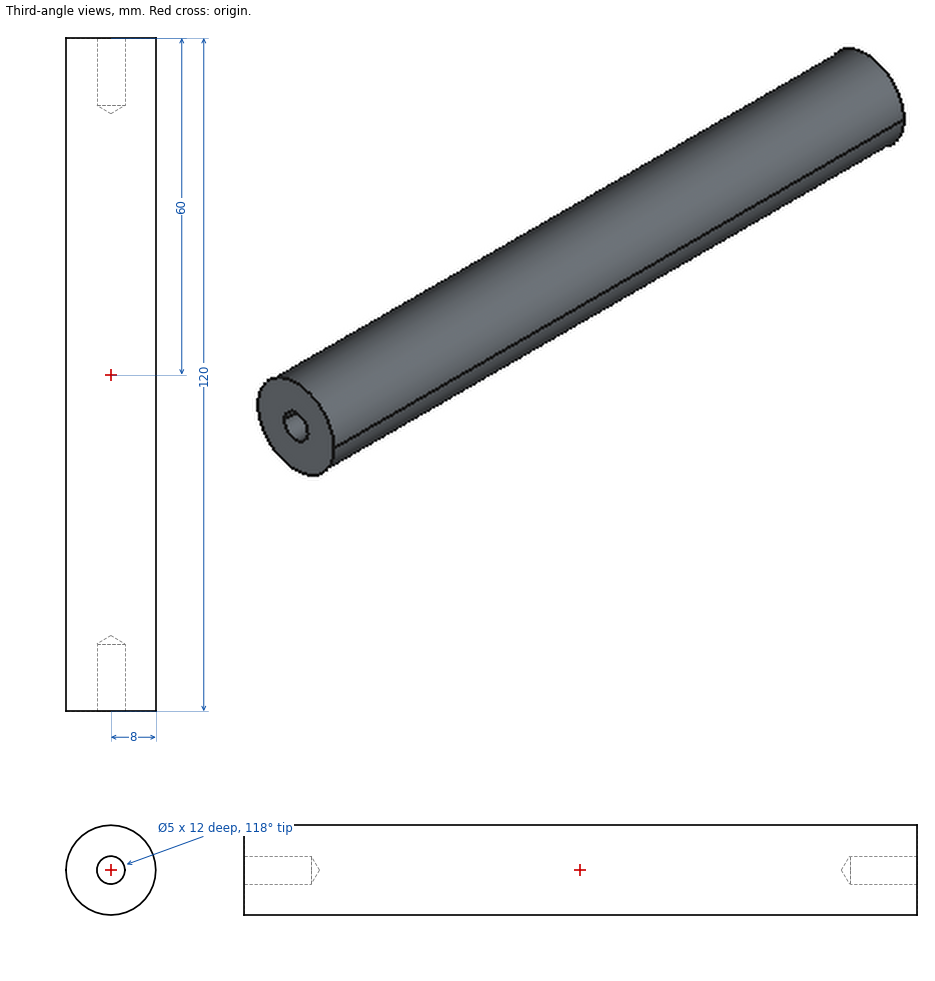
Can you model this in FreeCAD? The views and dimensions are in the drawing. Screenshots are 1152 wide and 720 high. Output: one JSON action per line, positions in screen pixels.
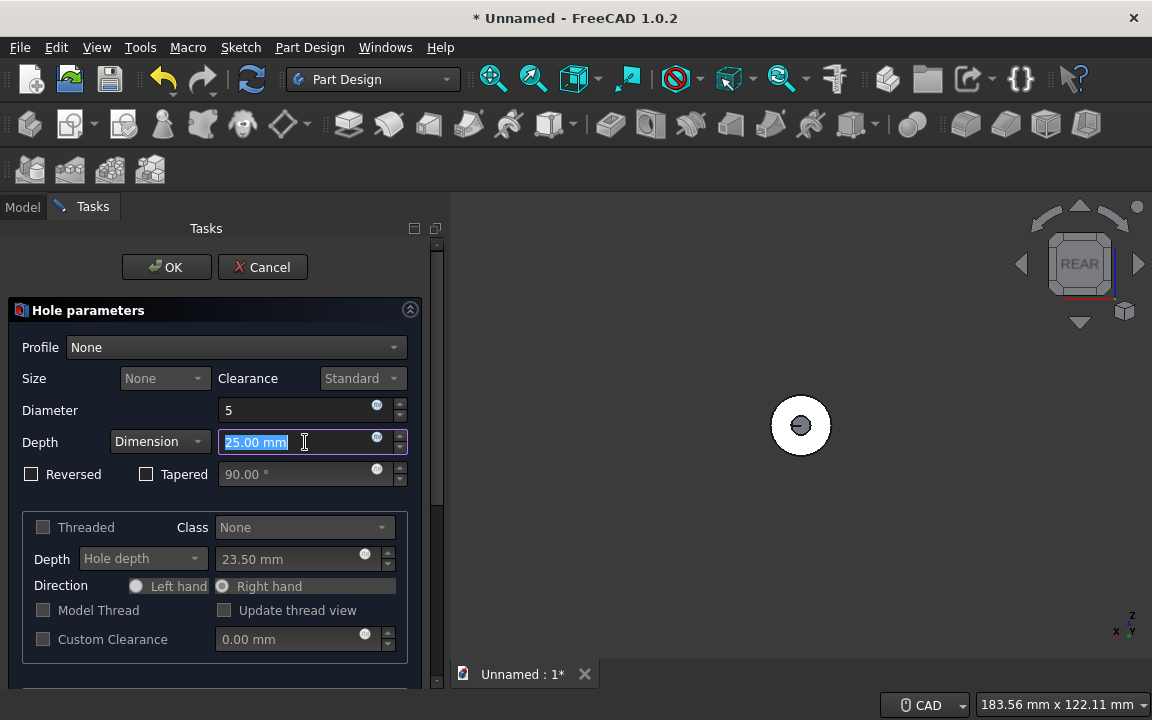
{"action": "type", "text": "12"}
{"action": "key", "text": "Tab"}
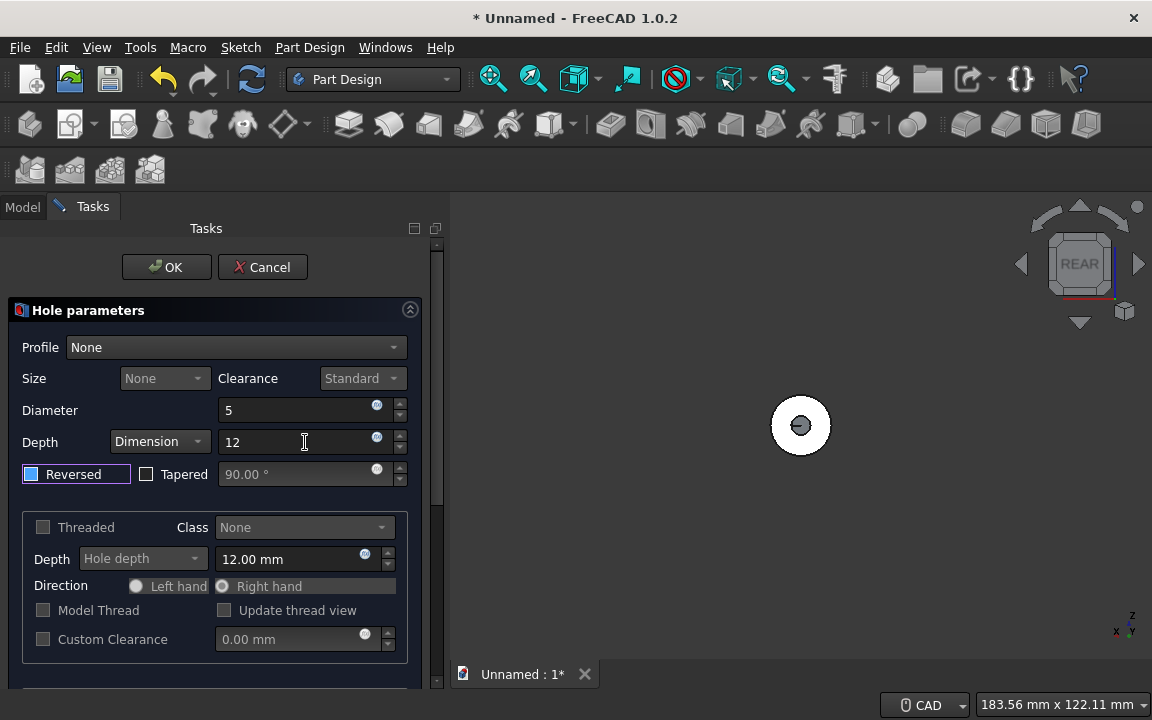
{"action": "left_click", "coordinate": [167, 267]}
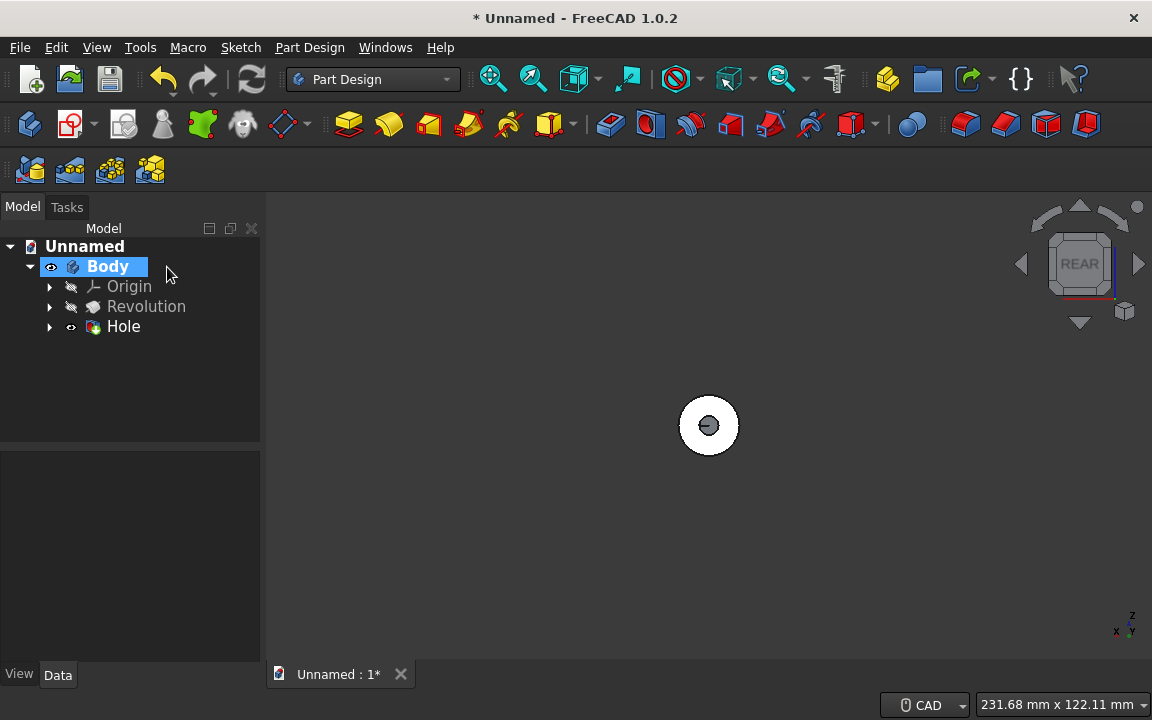
{"action": "left_click", "coordinate": [494, 80]}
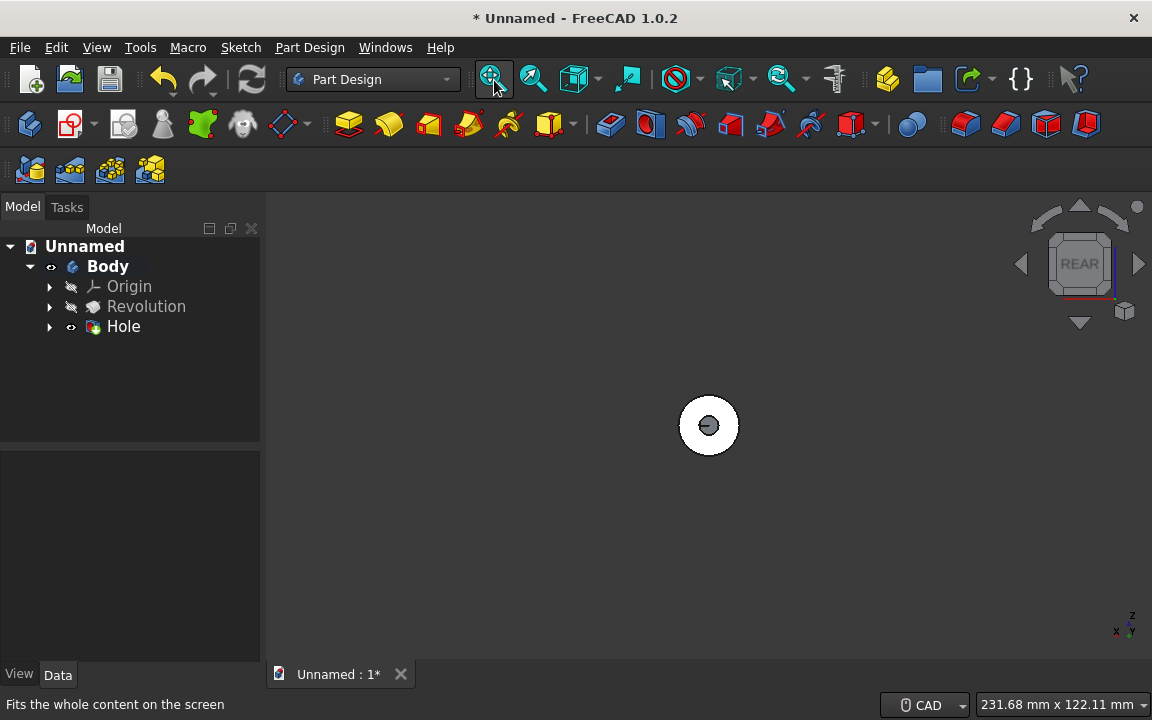
{"action": "key", "text": "0"}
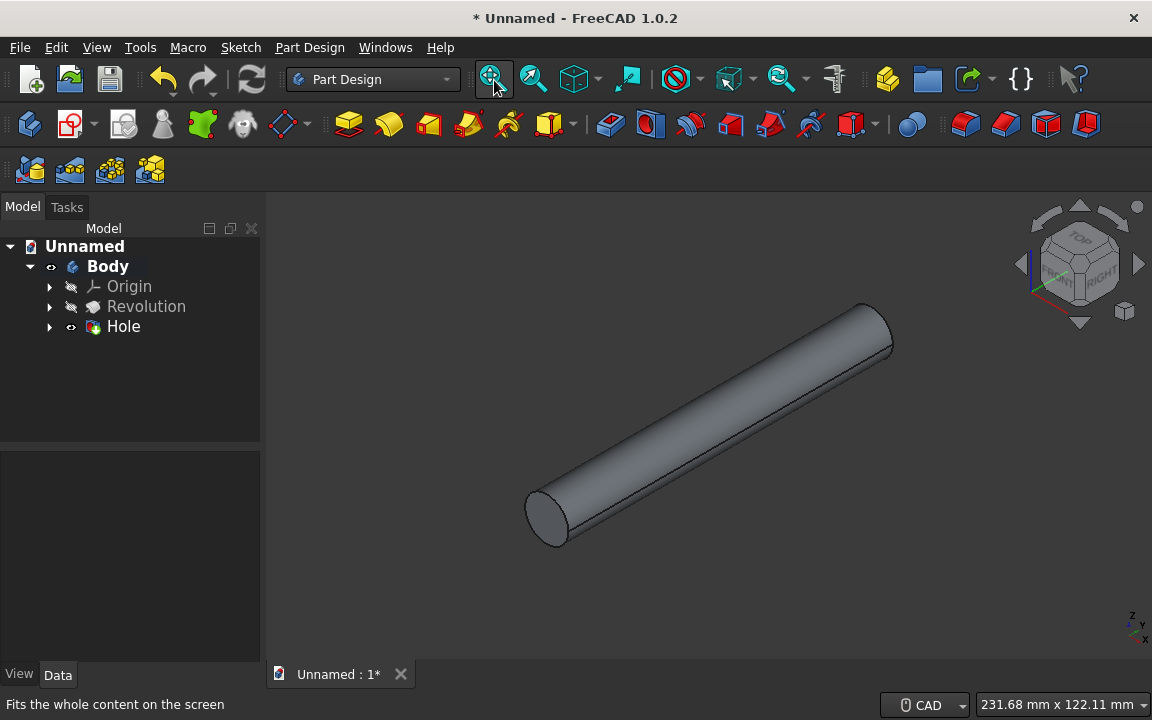
{"action": "left_click", "coordinate": [547, 518]}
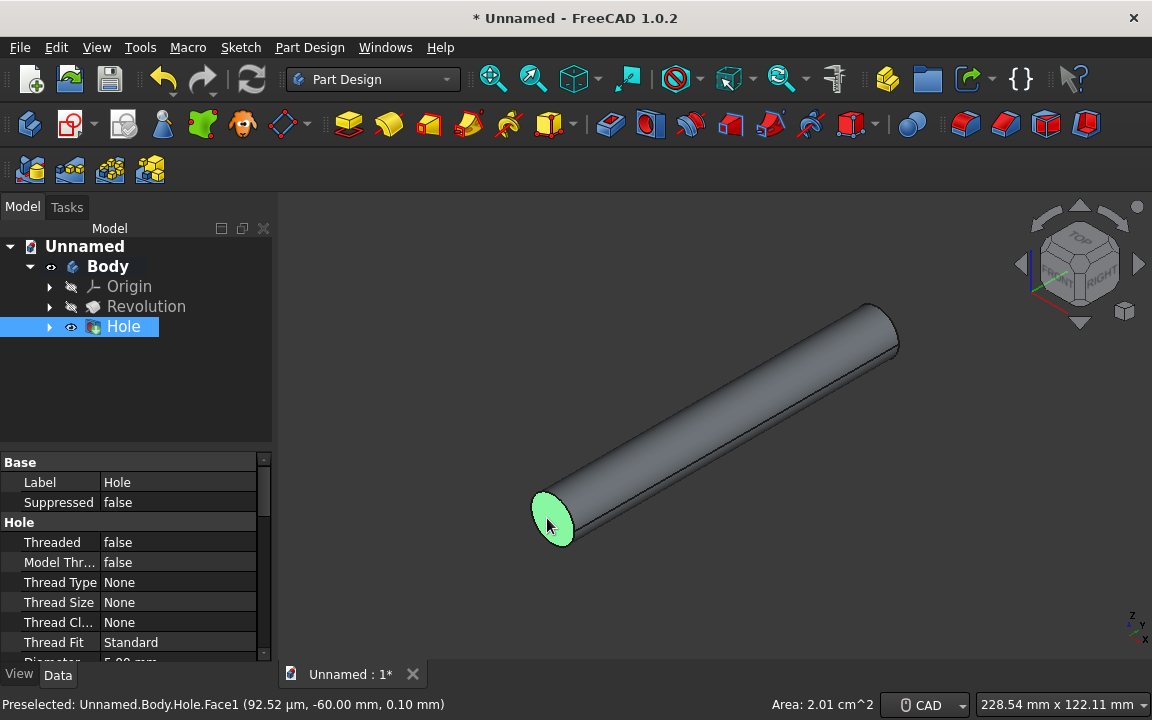
{"action": "left_click", "coordinate": [70, 124]}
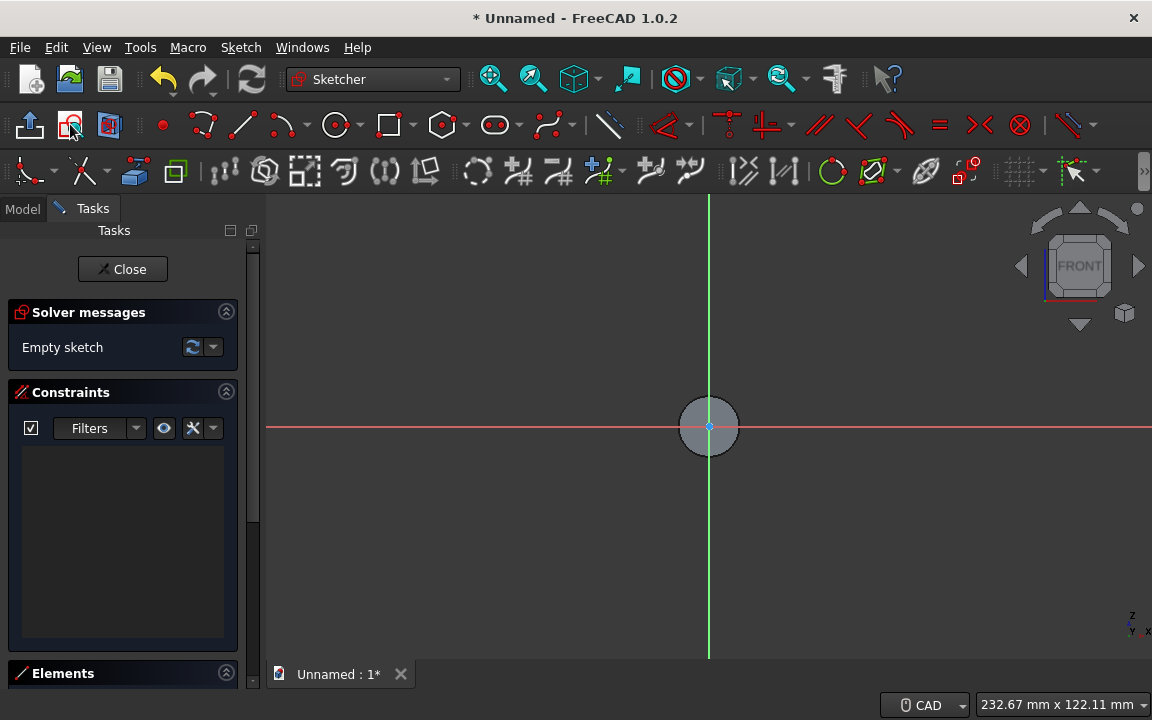
{"action": "scroll", "coordinate": [713, 427], "scroll_direction": "up", "scroll_amount": 14}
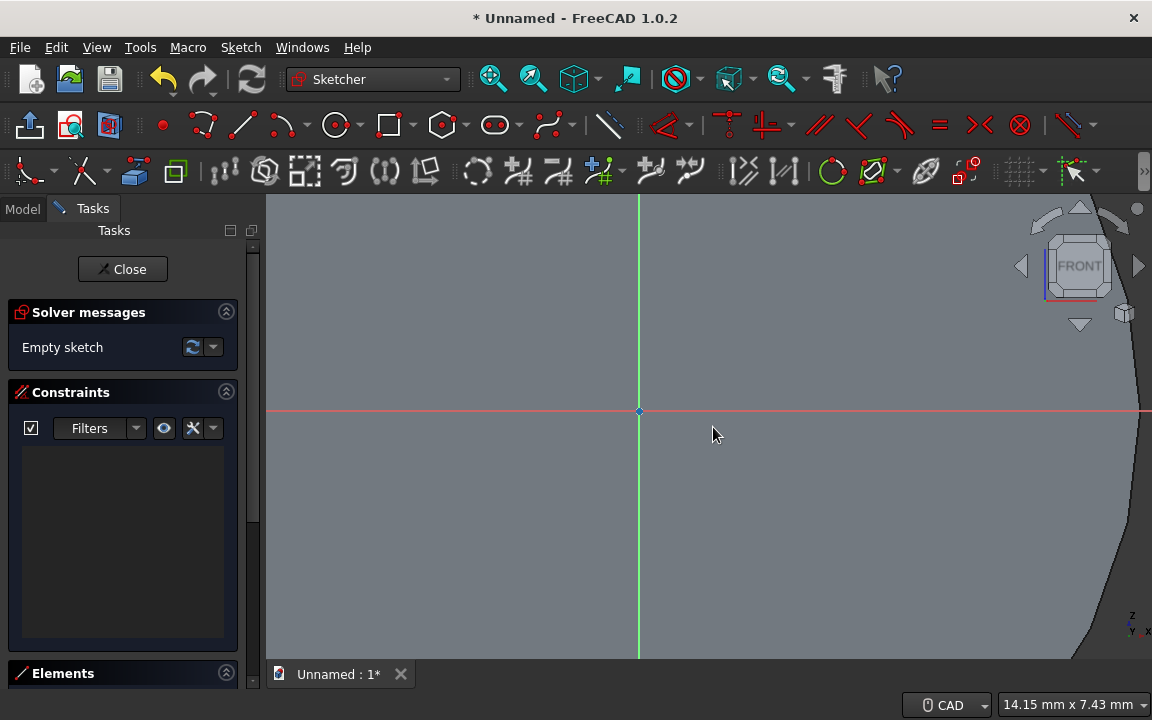
{"action": "key", "text": "g c"}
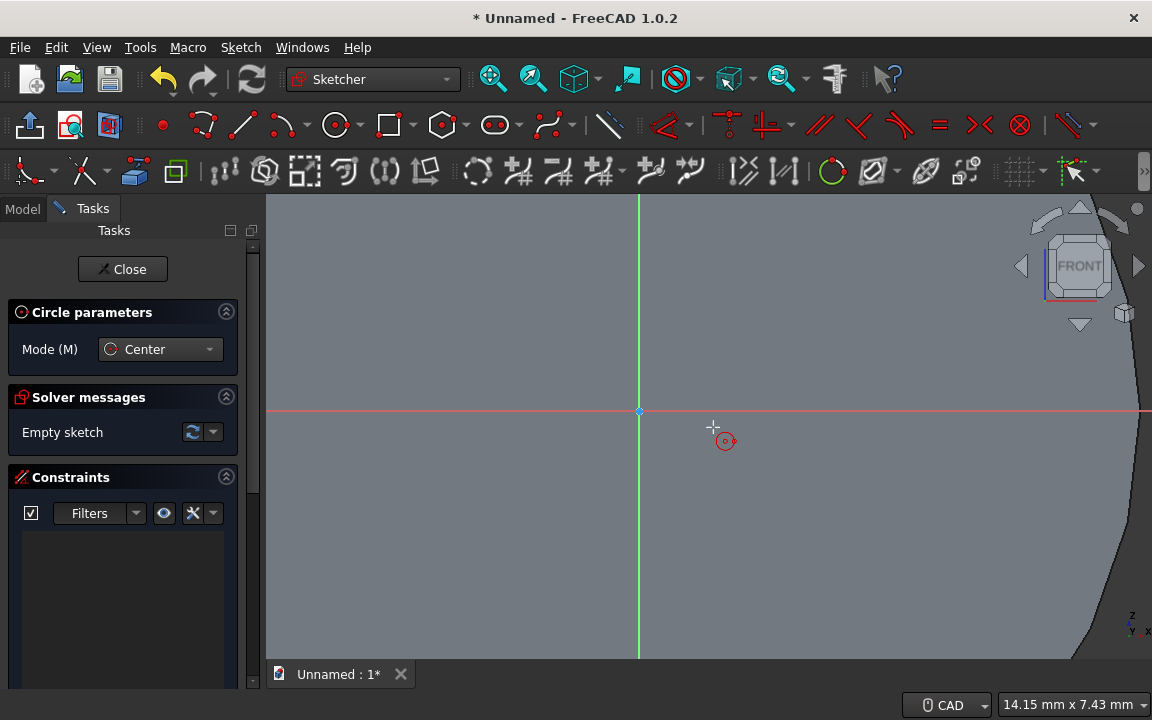
{"action": "left_click", "coordinate": [639, 411]}
{"action": "left_click", "coordinate": [750, 300]}
{"action": "key", "text": "Escape"}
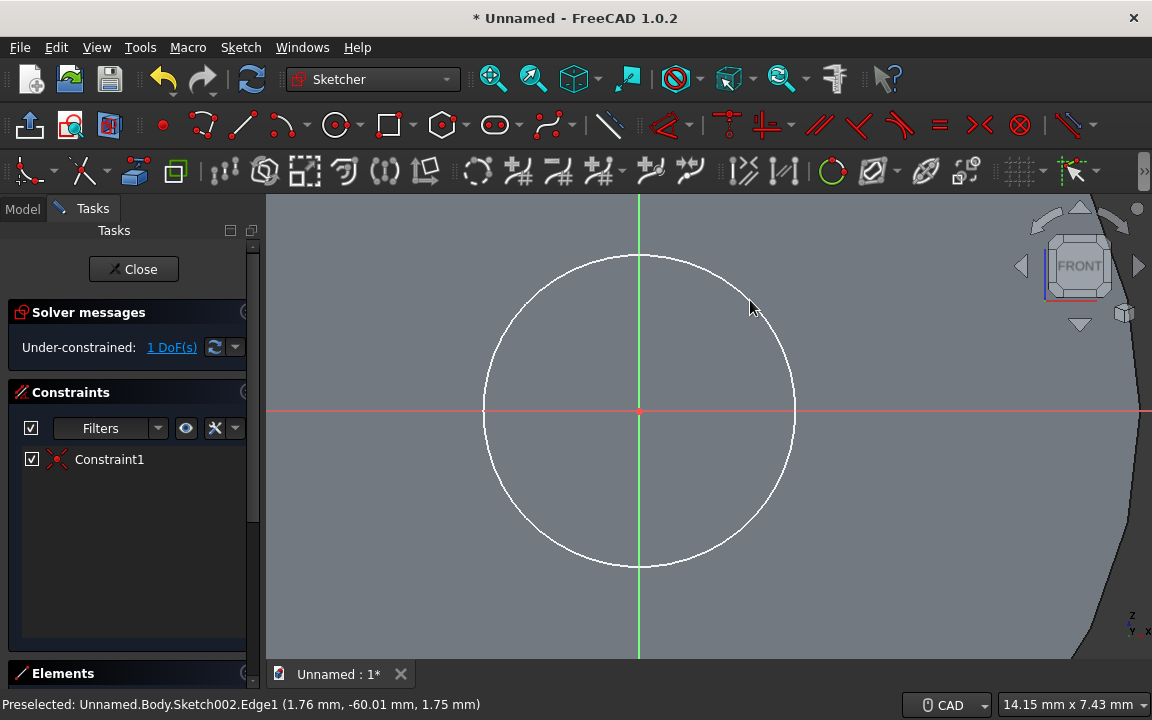
{"action": "left_click", "coordinate": [749, 300]}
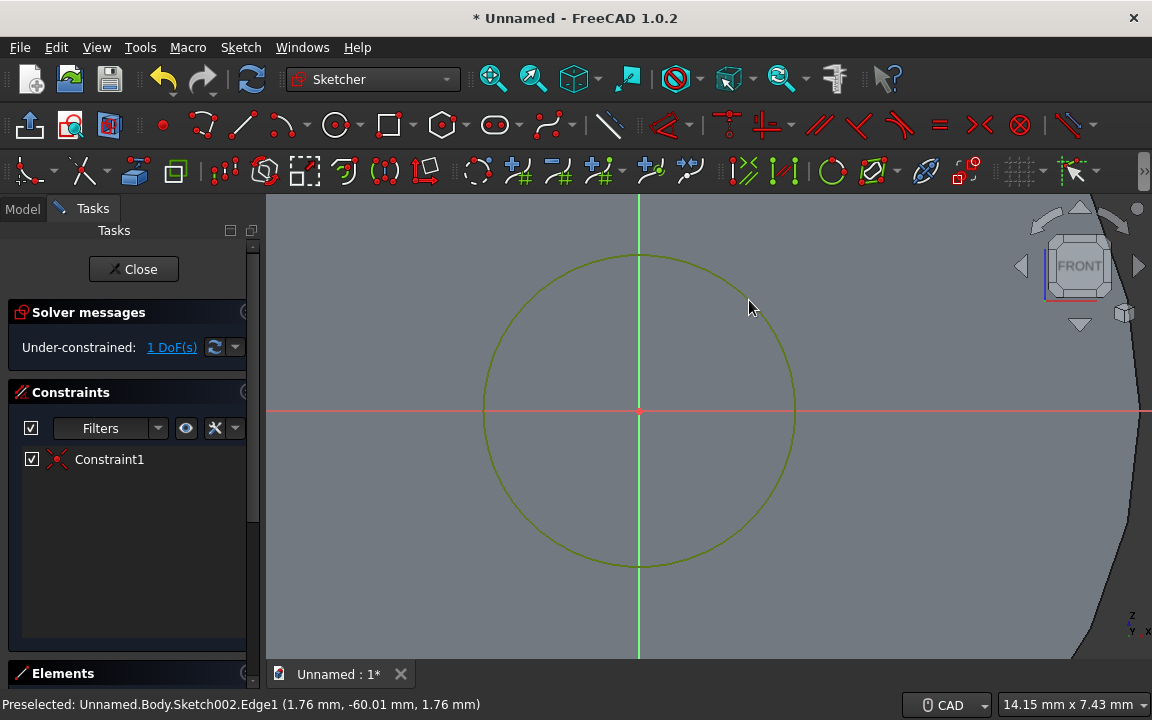
{"action": "left_click", "coordinate": [692, 126]}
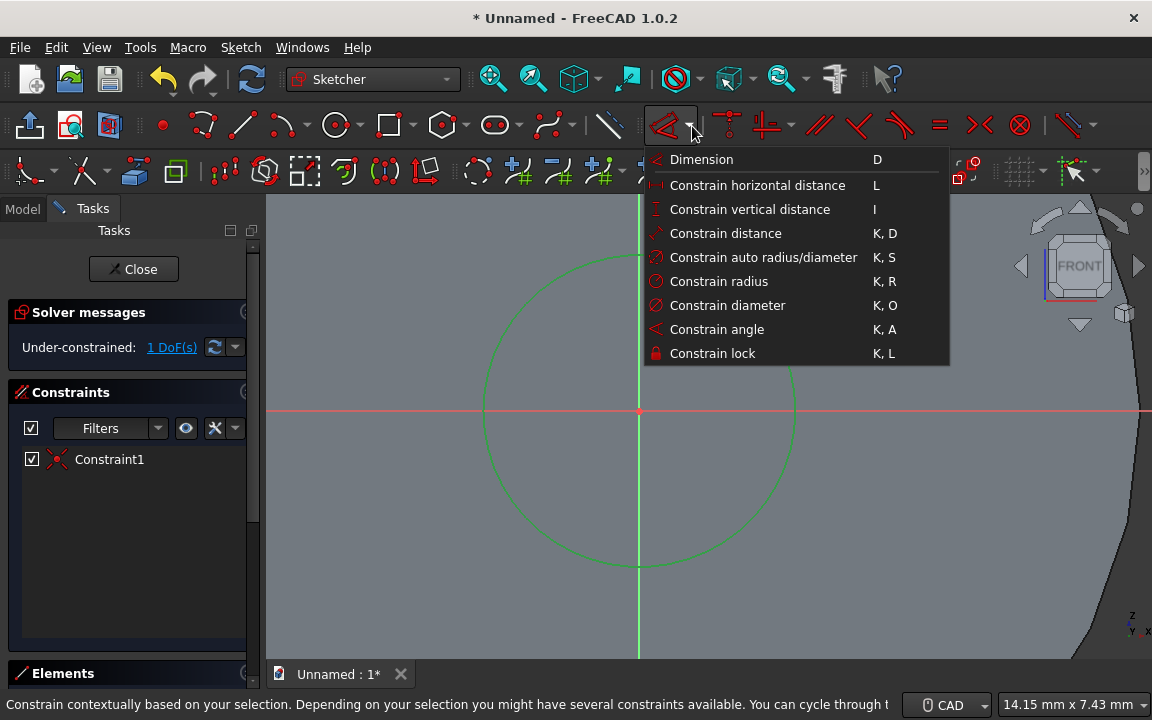
{"action": "left_click", "coordinate": [797, 305]}